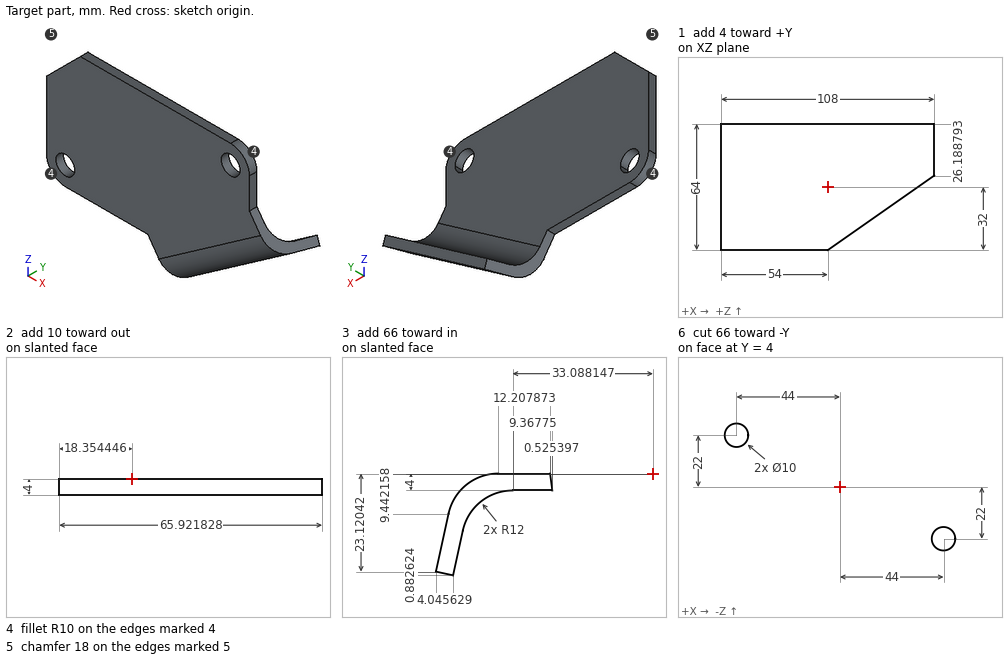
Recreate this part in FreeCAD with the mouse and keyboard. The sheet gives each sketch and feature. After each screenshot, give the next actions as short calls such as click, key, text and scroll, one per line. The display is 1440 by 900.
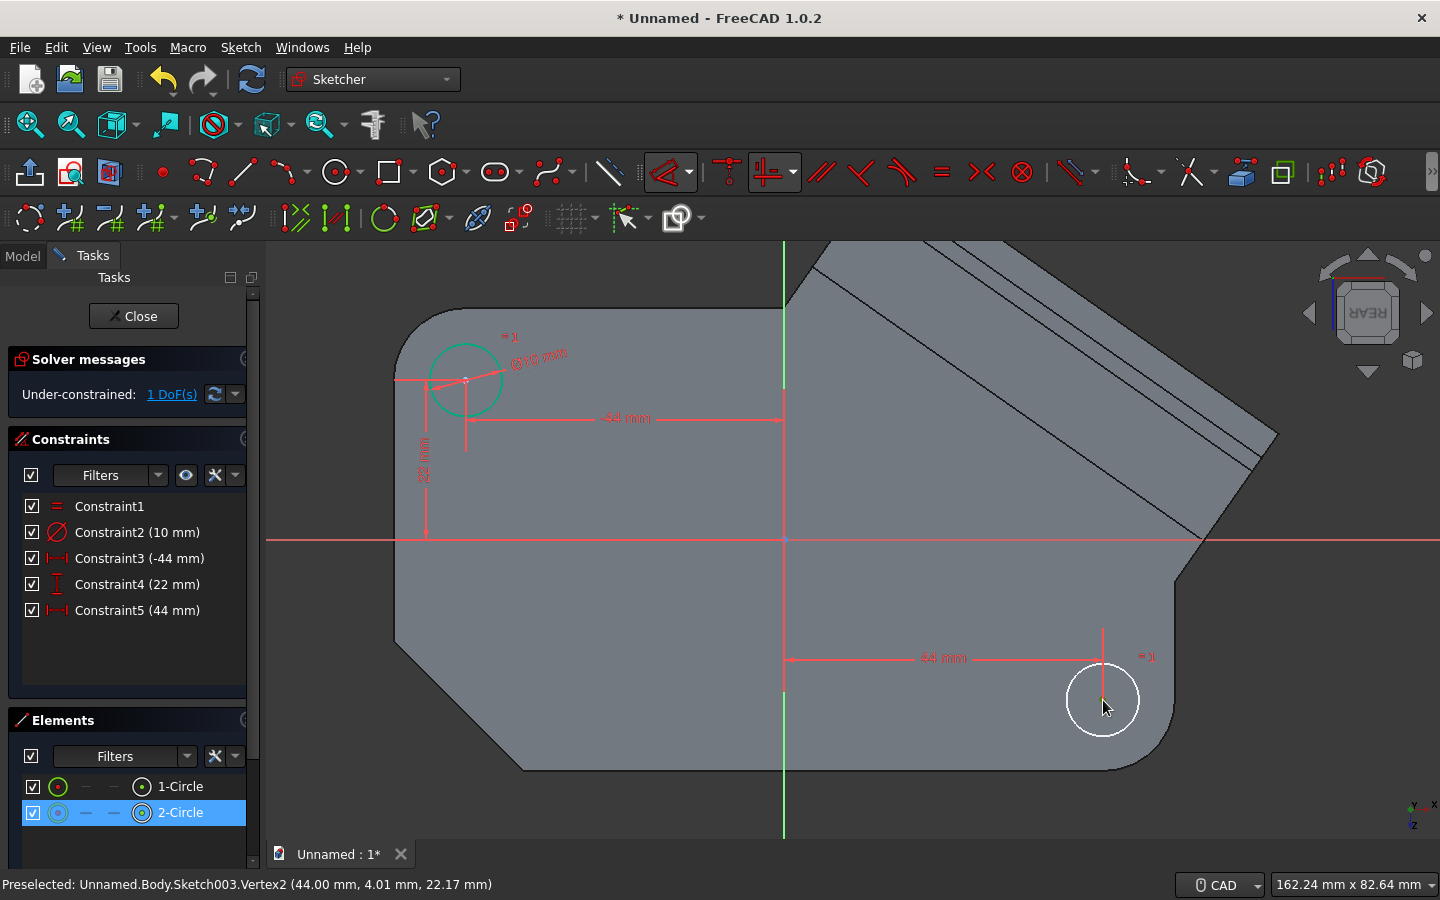
click(692, 172)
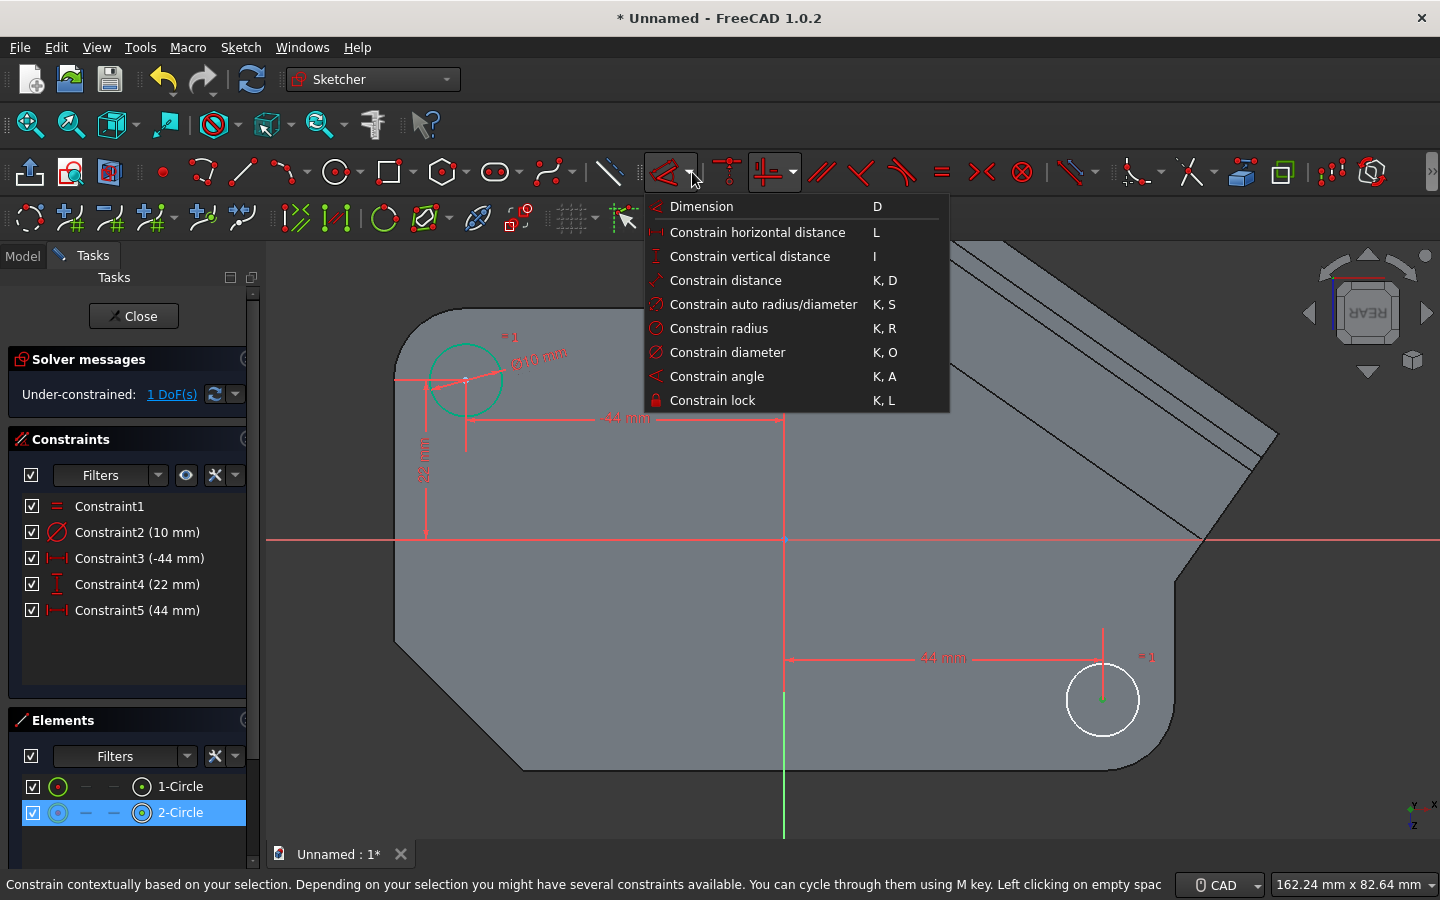
click(797, 256)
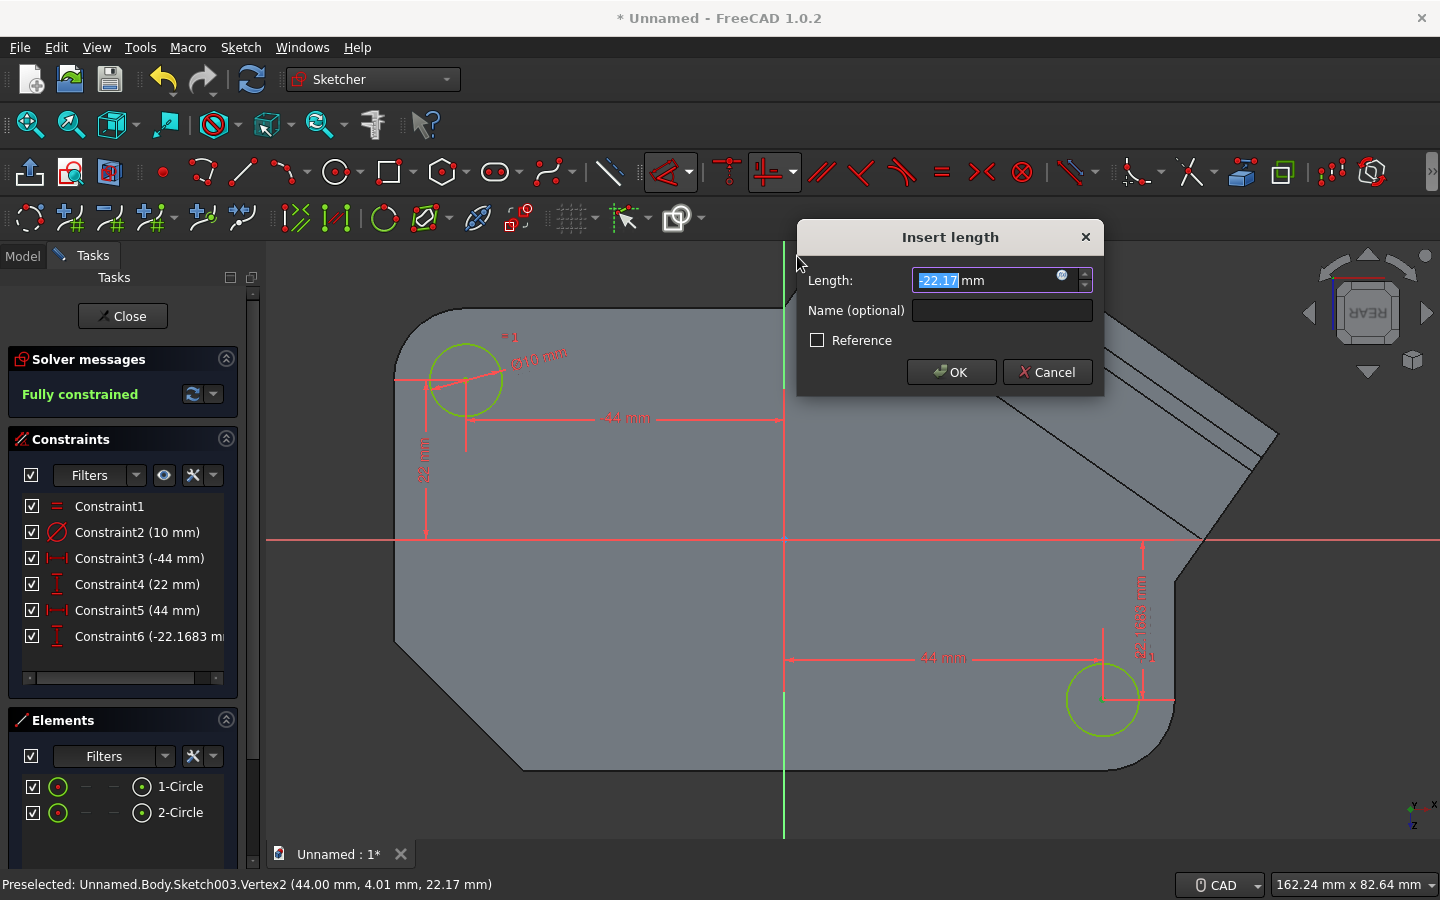
text(-22)
key(Return)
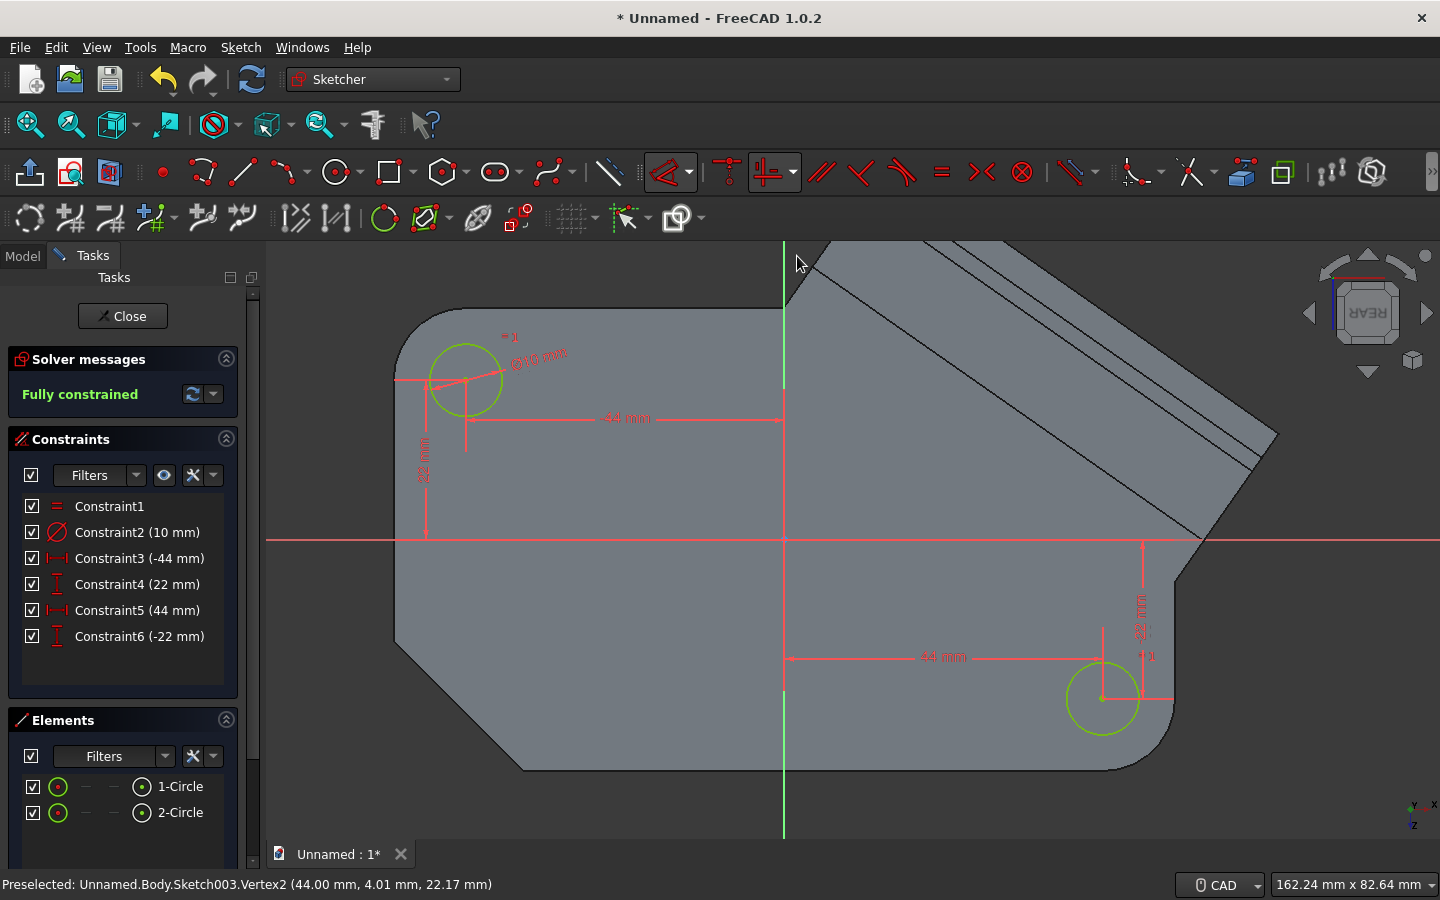
click(123, 316)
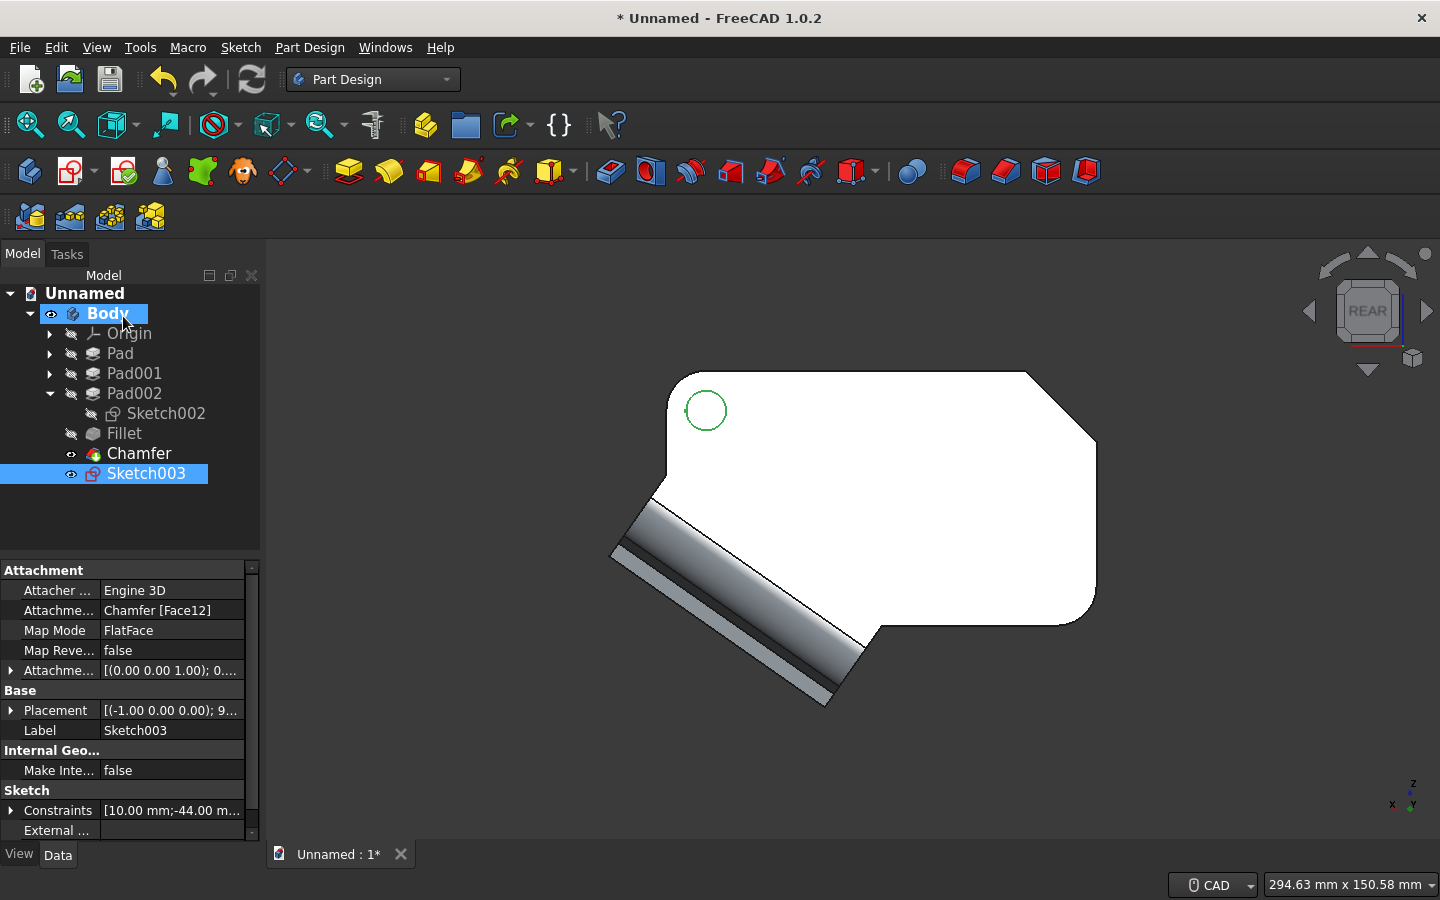
click(612, 172)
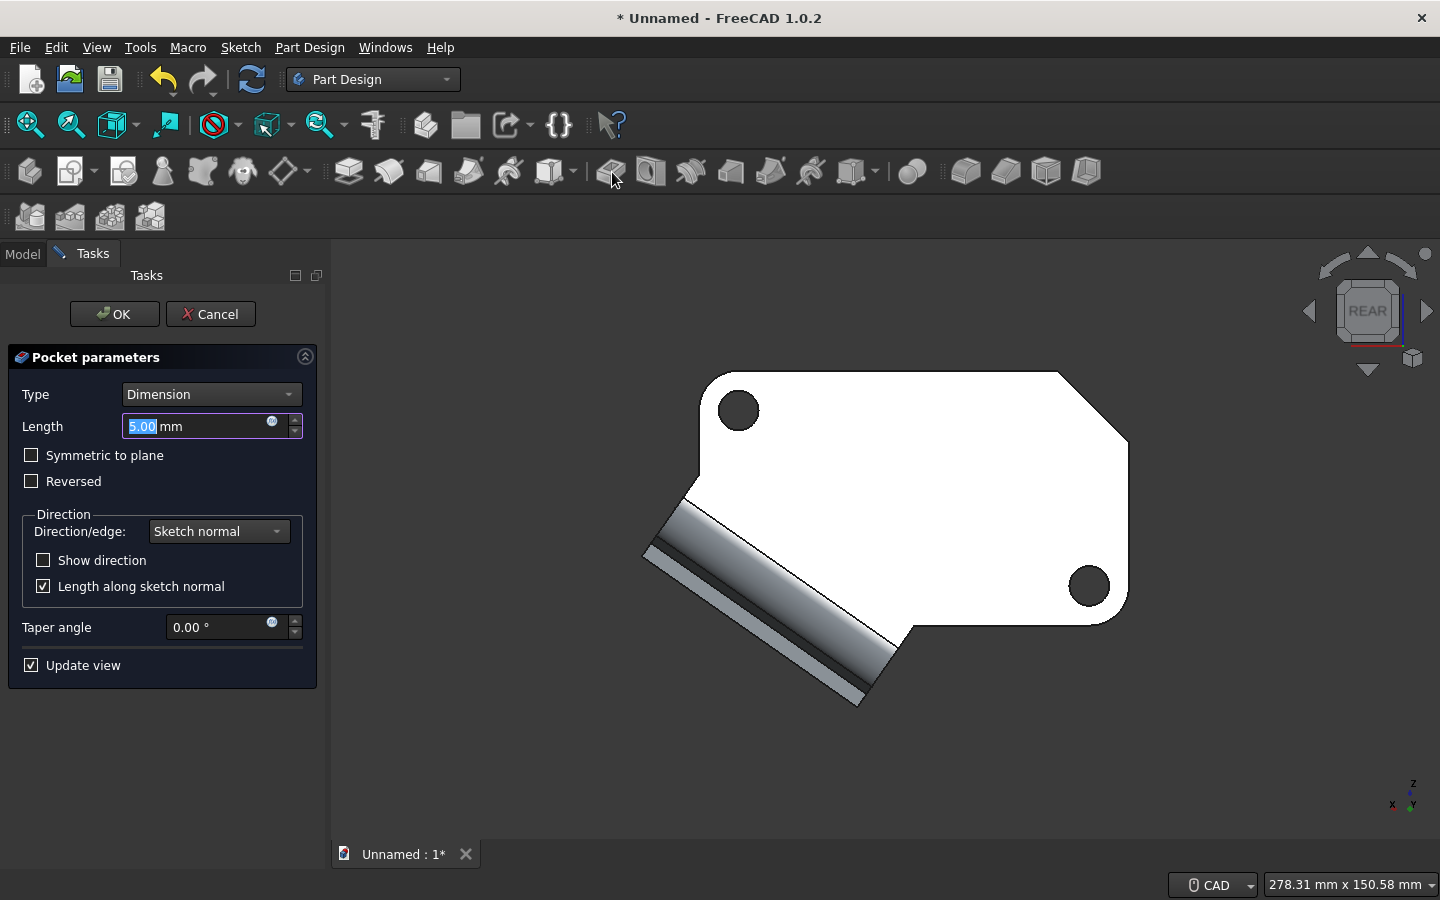
text(66)
key(Tab)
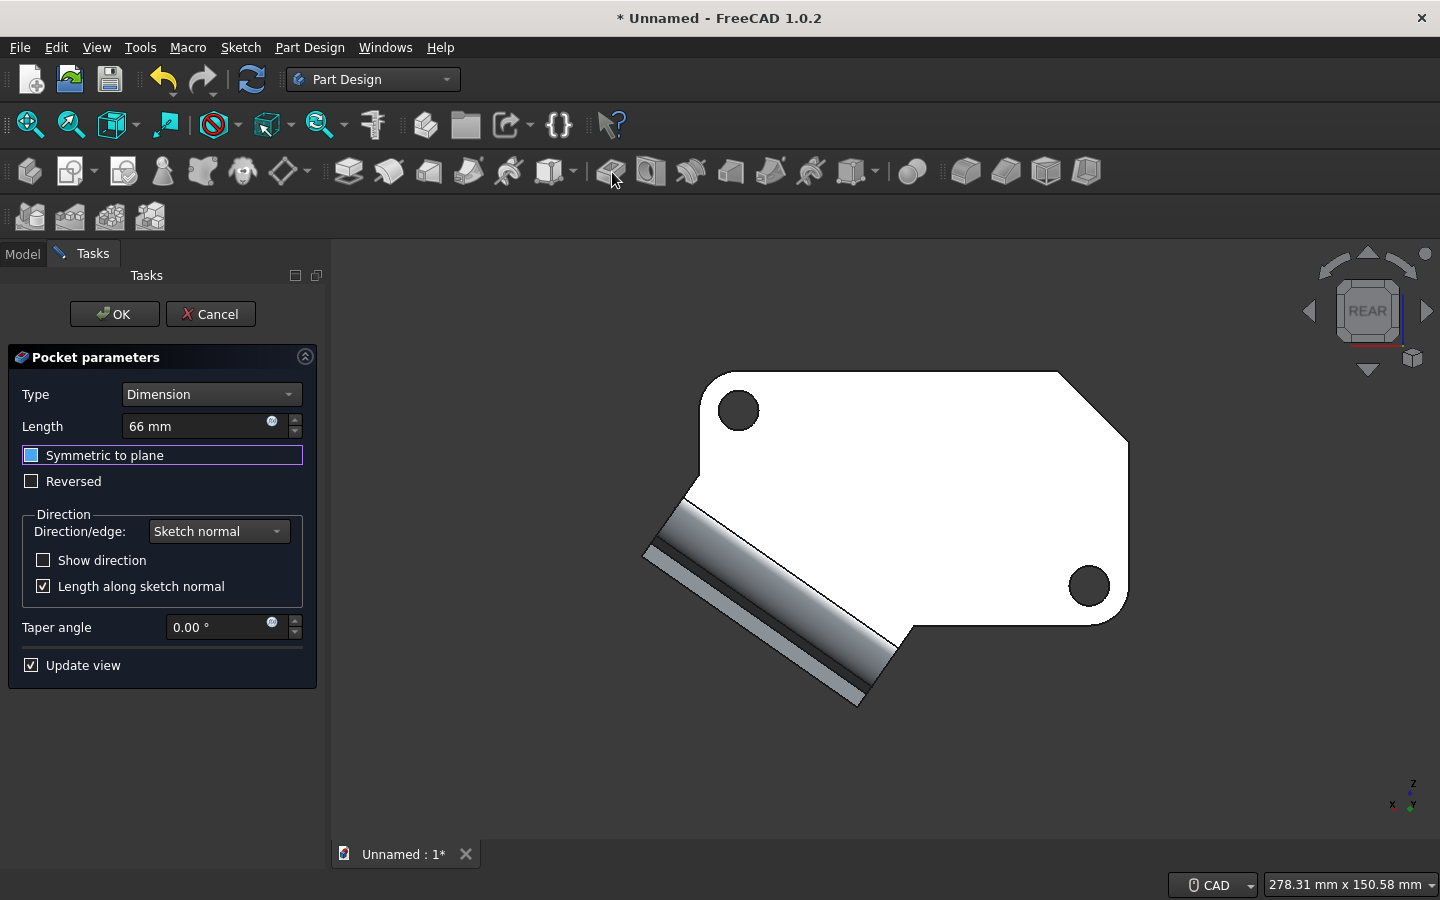
click(115, 314)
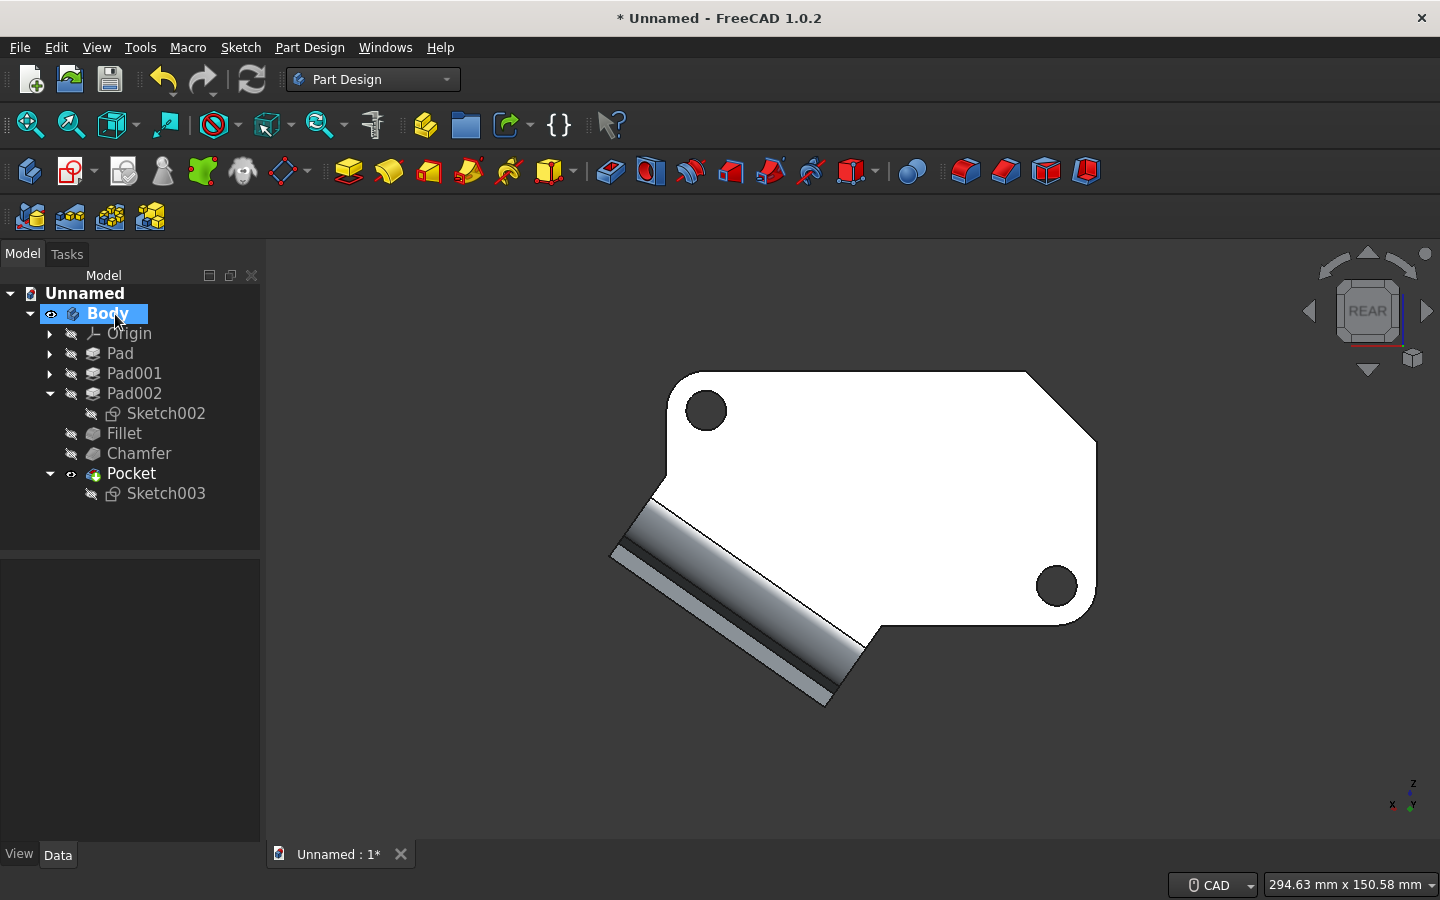
key(0)